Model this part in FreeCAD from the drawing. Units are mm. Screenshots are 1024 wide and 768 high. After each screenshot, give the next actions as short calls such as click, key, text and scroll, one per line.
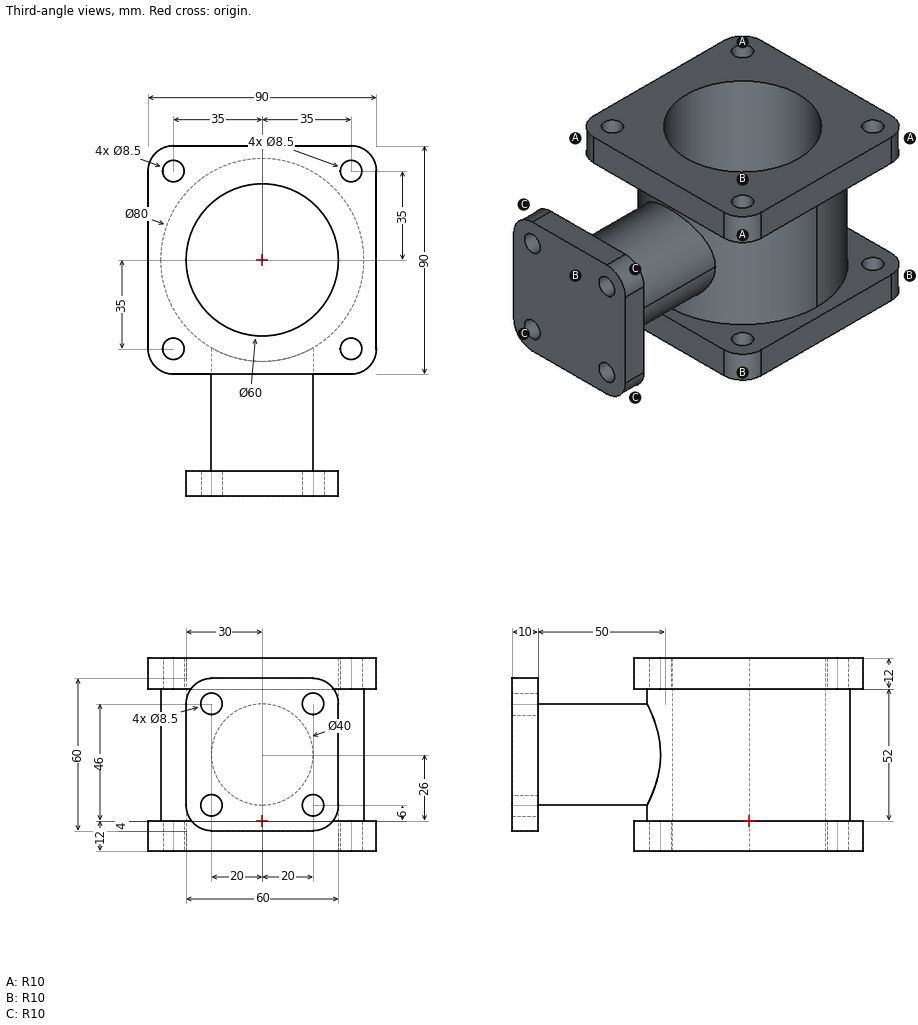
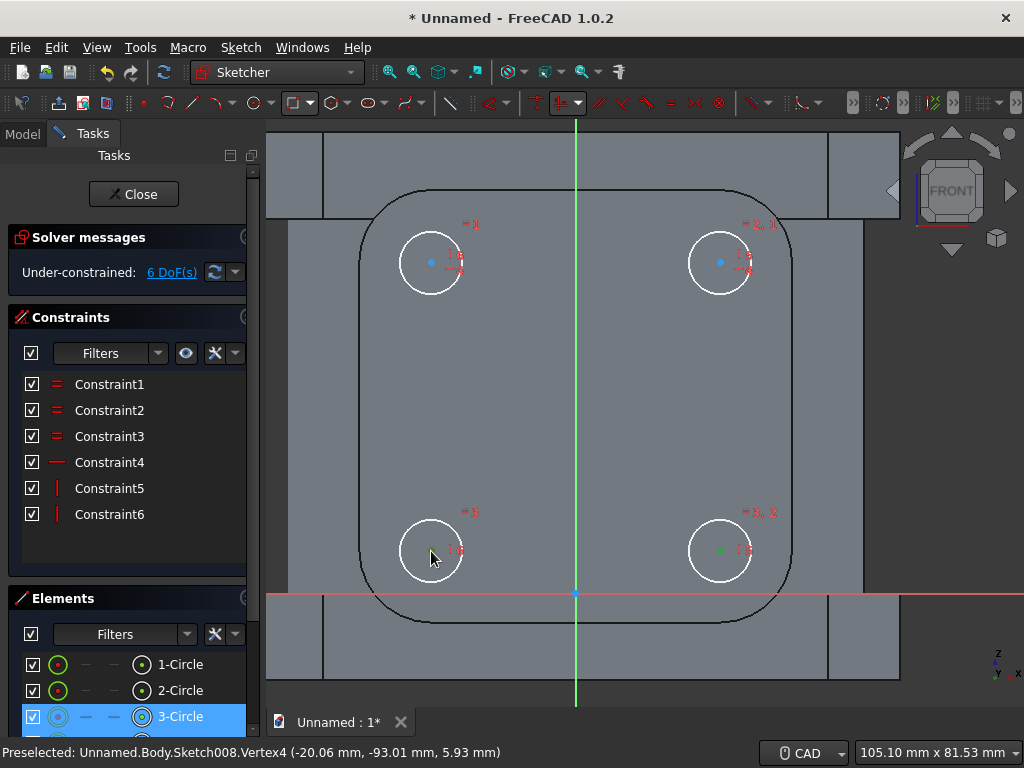
key(h)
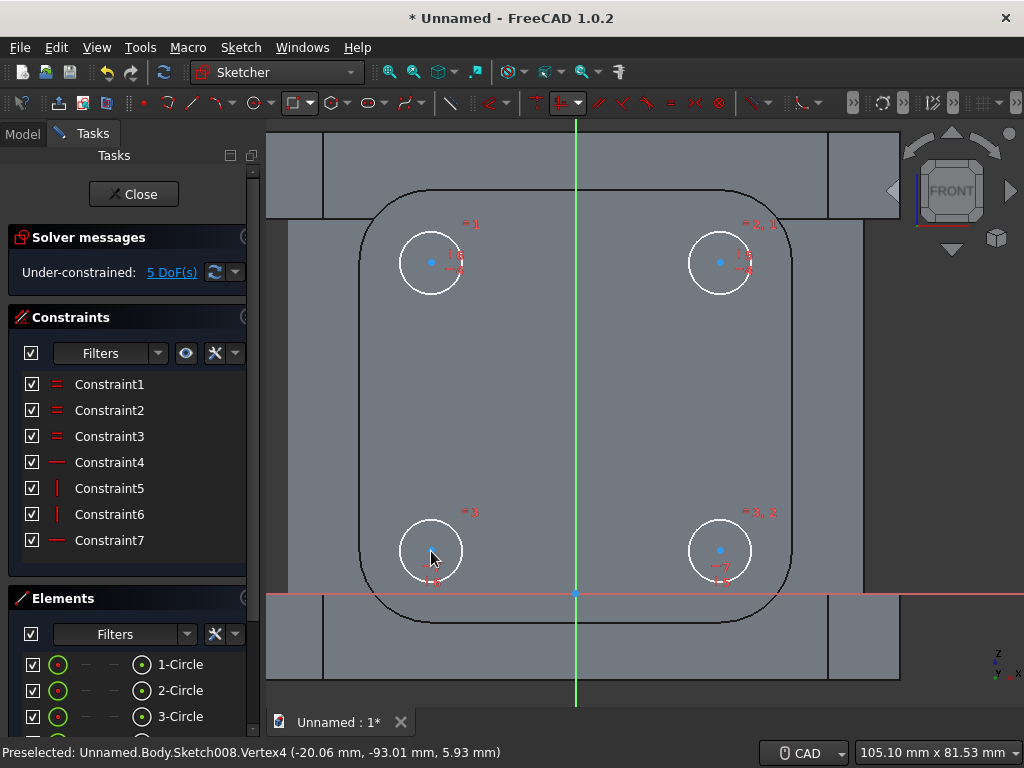
click(490, 104)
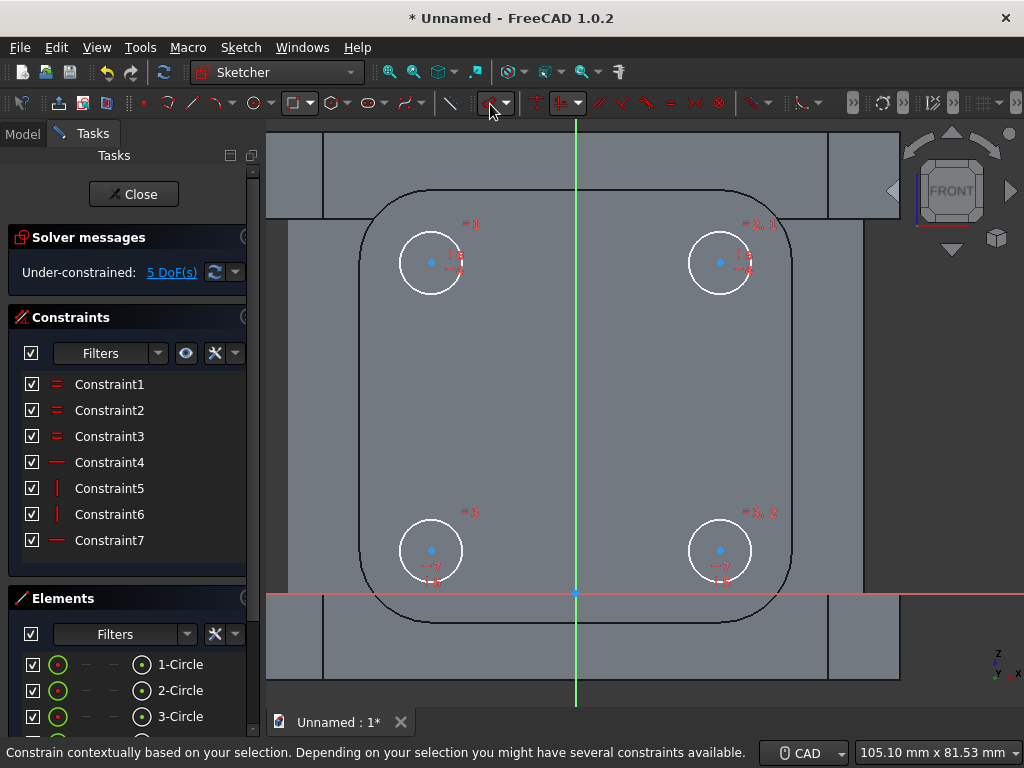
click(453, 241)
click(476, 218)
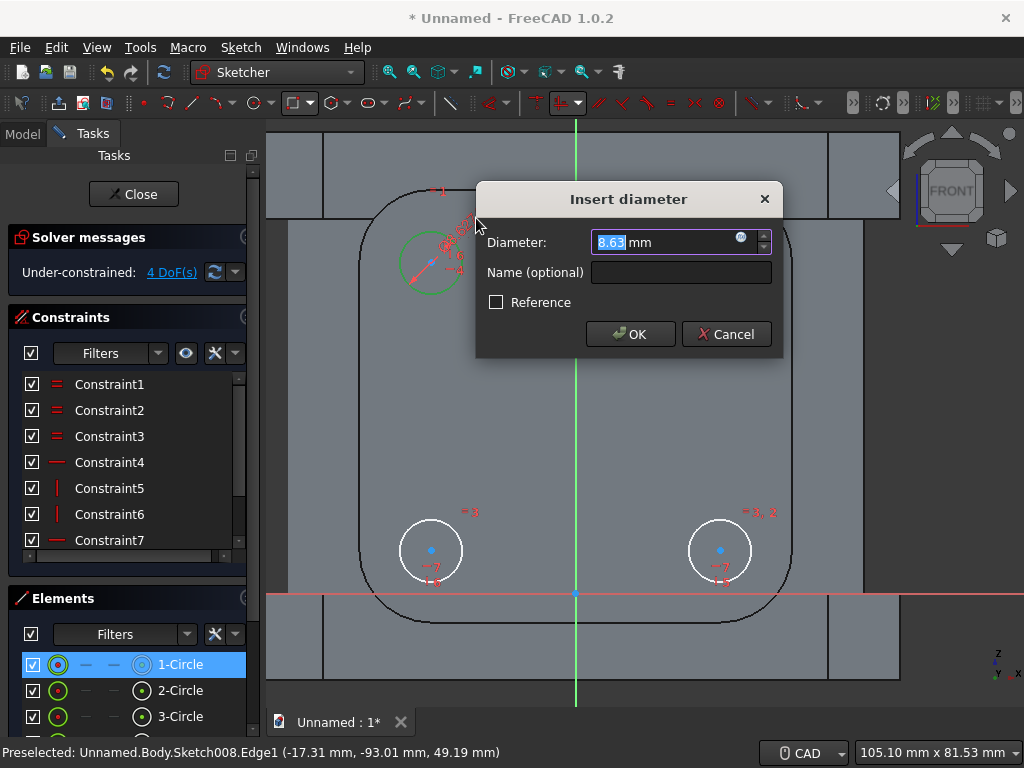
text(8.5)
key(Return)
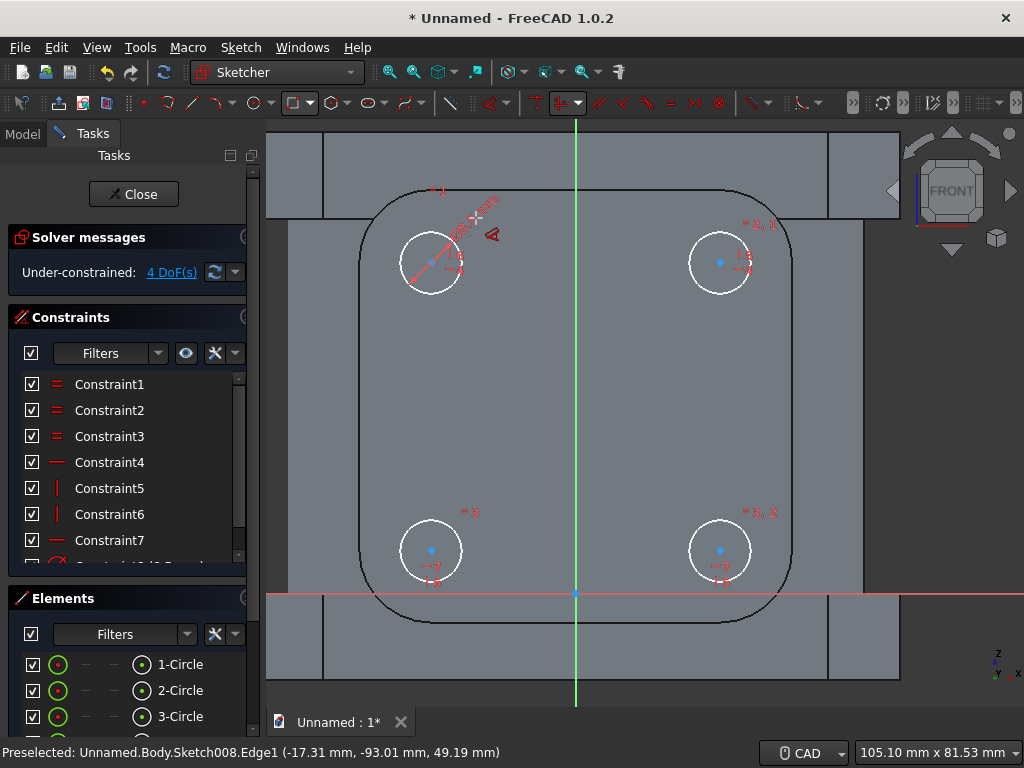
click(720, 551)
click(542, 572)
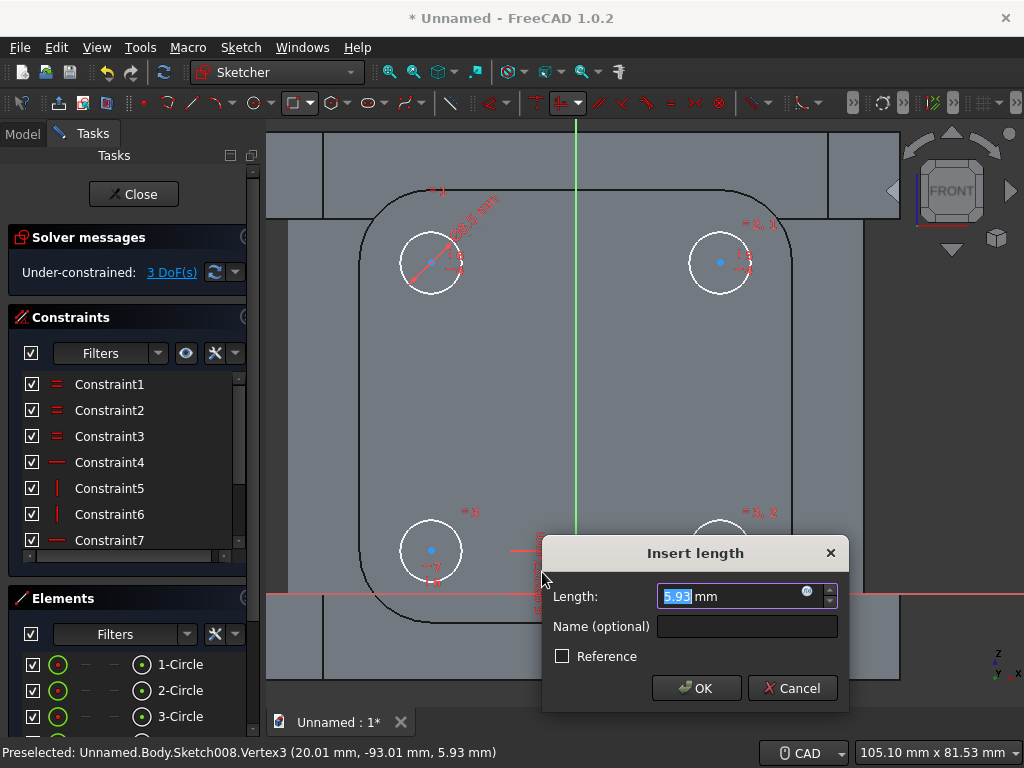
text(6)
key(Return)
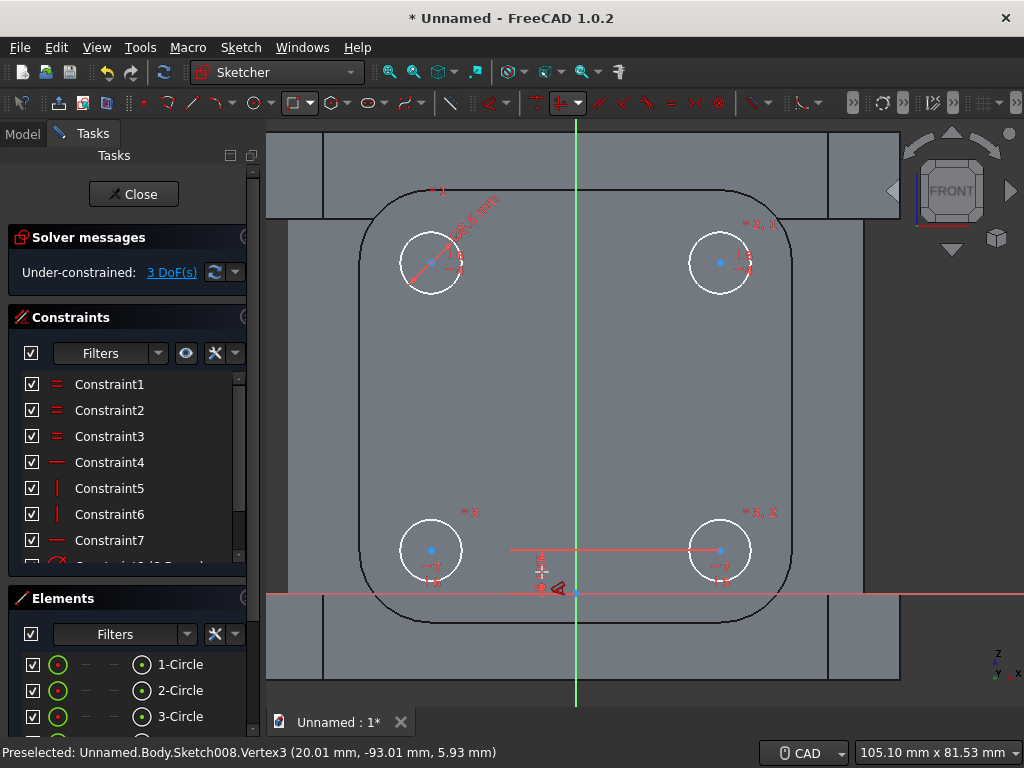
click(431, 263)
click(503, 628)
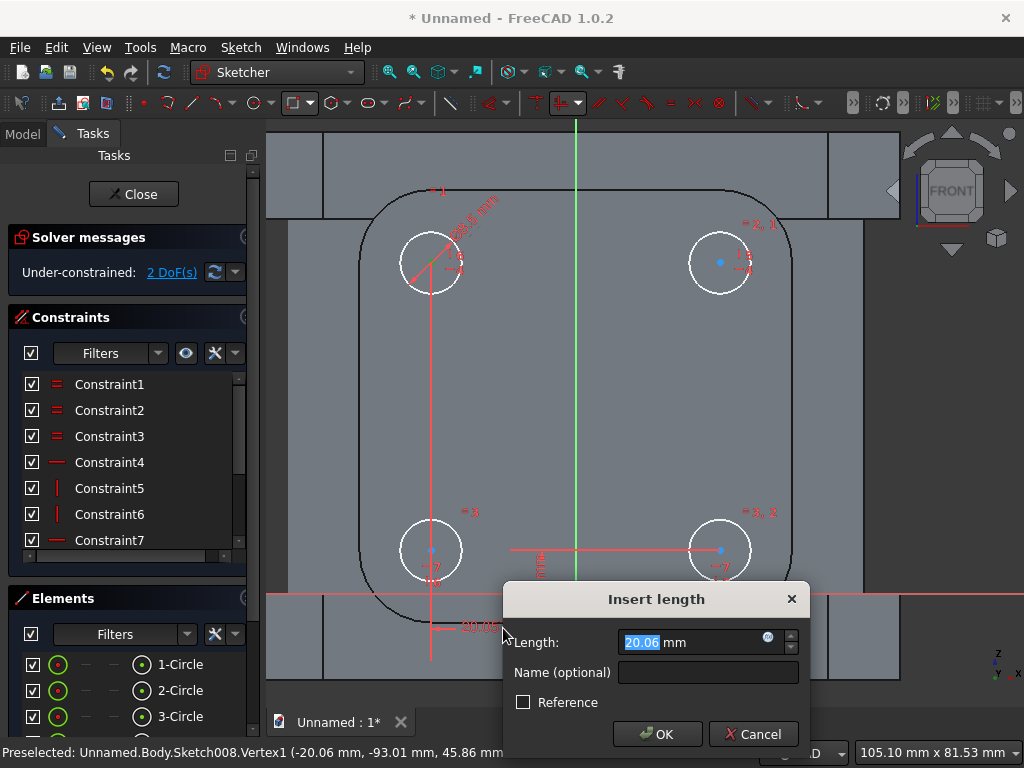
text(20)
key(Return)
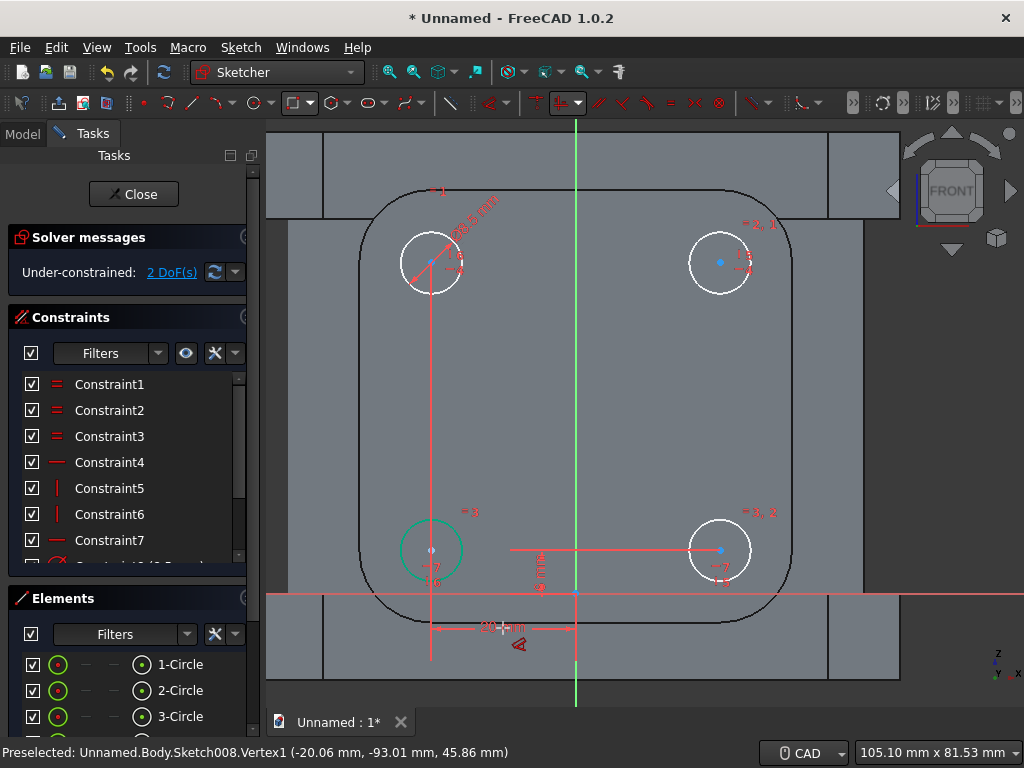
click(431, 263)
click(397, 428)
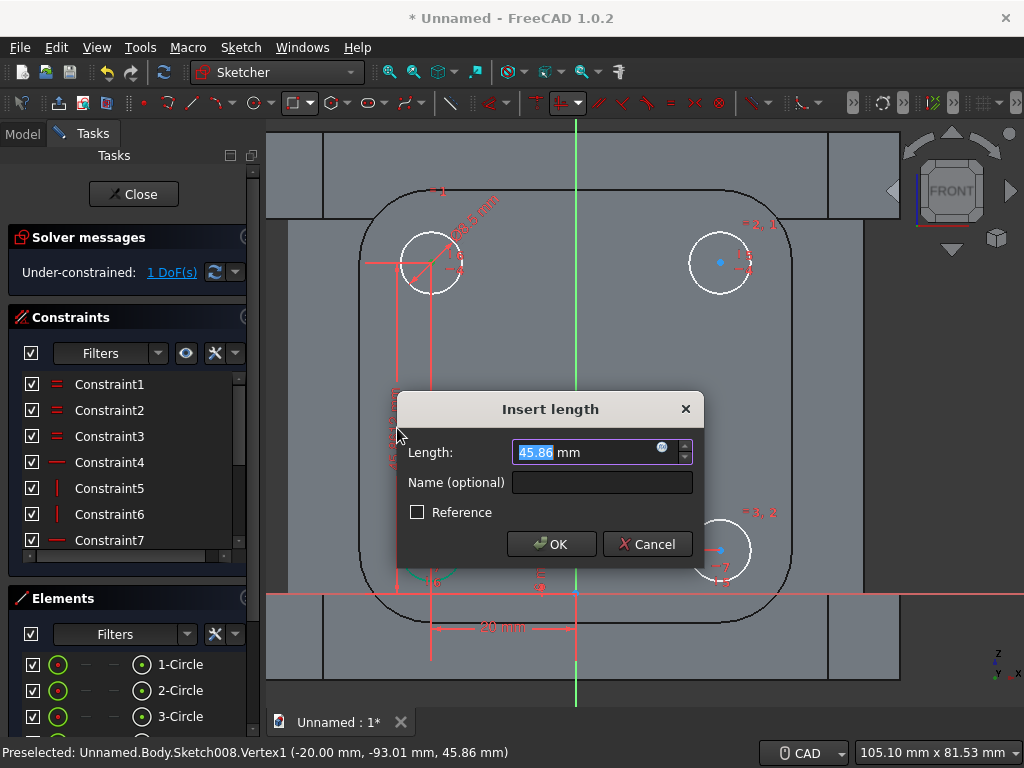
text(46)
key(Return)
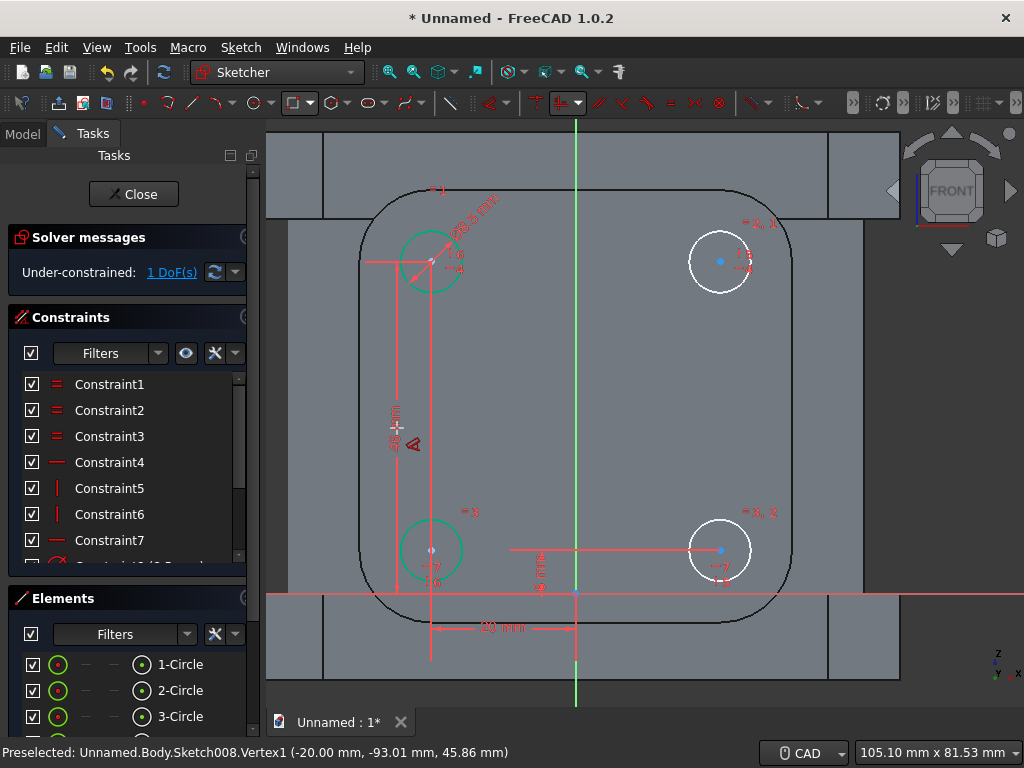
click(720, 262)
click(648, 628)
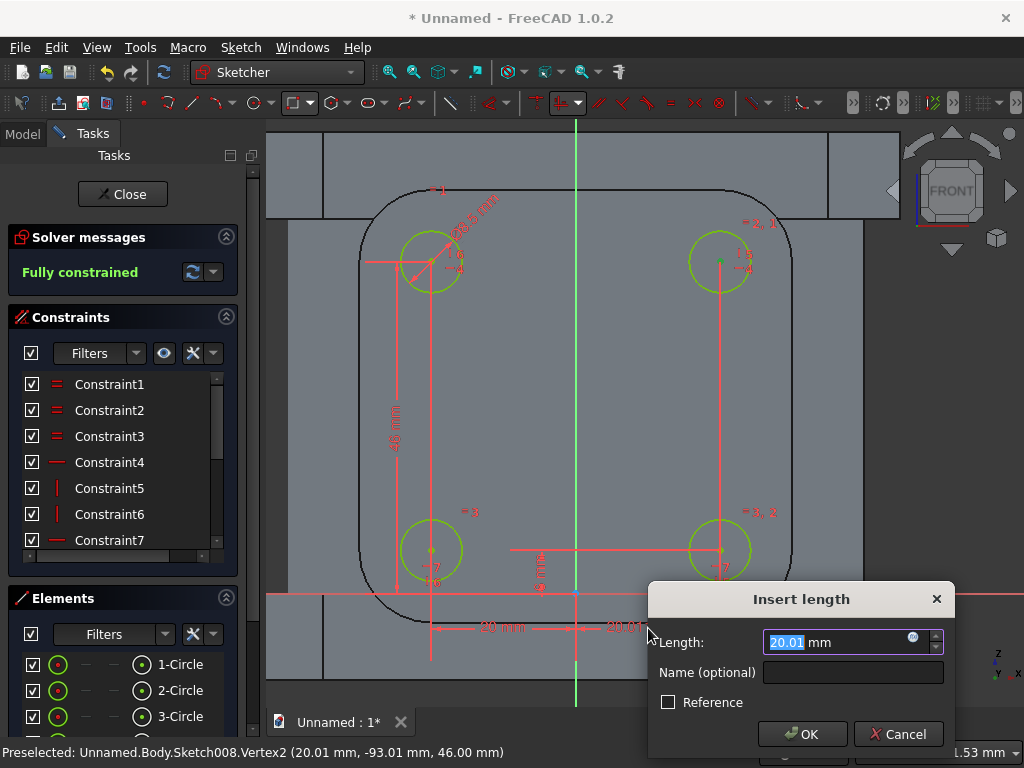
text(20)
key(Return)
key(Escape)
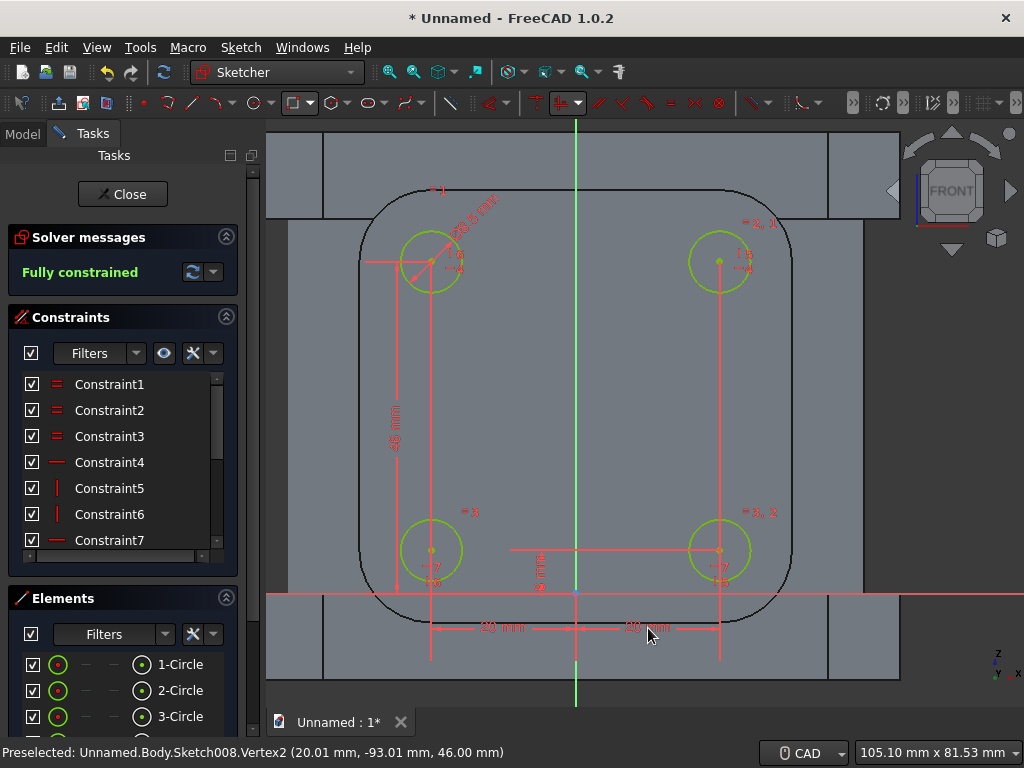
click(123, 194)